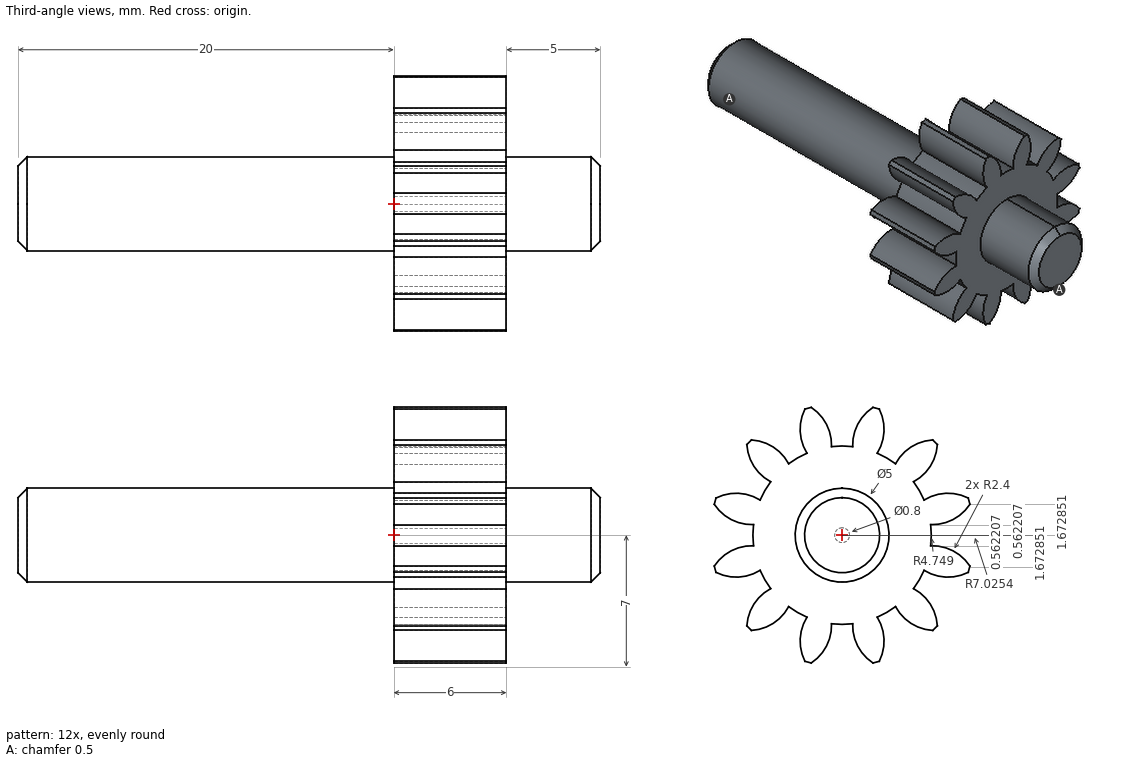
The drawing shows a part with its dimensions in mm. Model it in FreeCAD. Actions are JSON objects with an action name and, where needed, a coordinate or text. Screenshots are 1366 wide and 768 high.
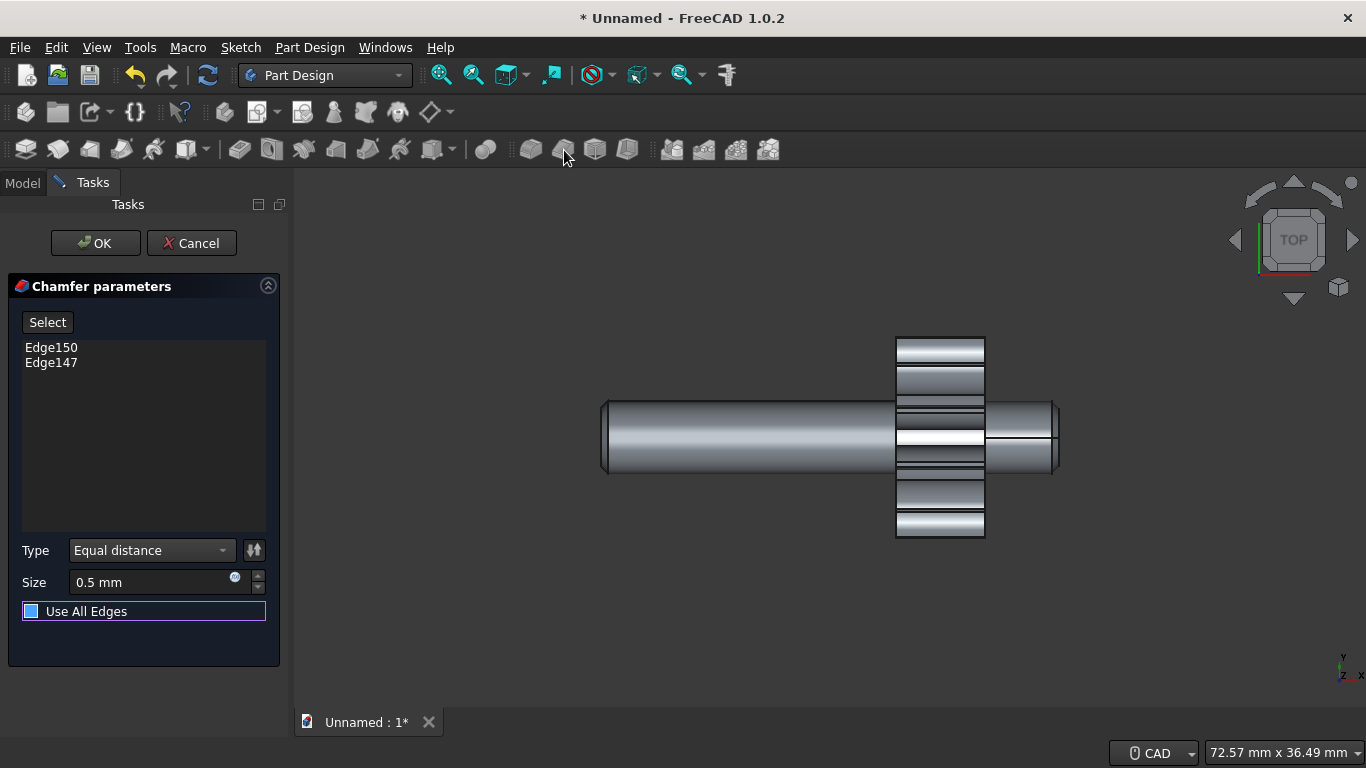
{"action": "left_click", "coordinate": [96, 243]}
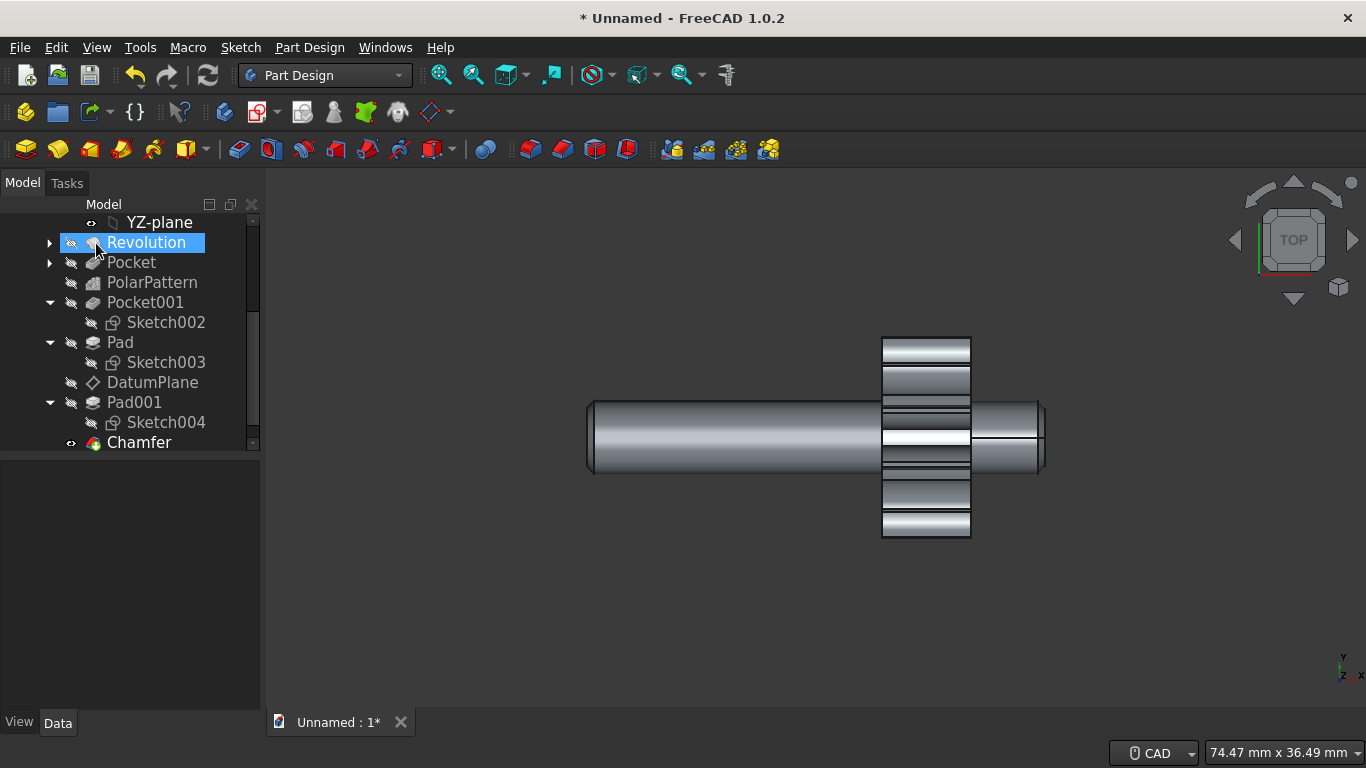
{"action": "key", "text": "0"}